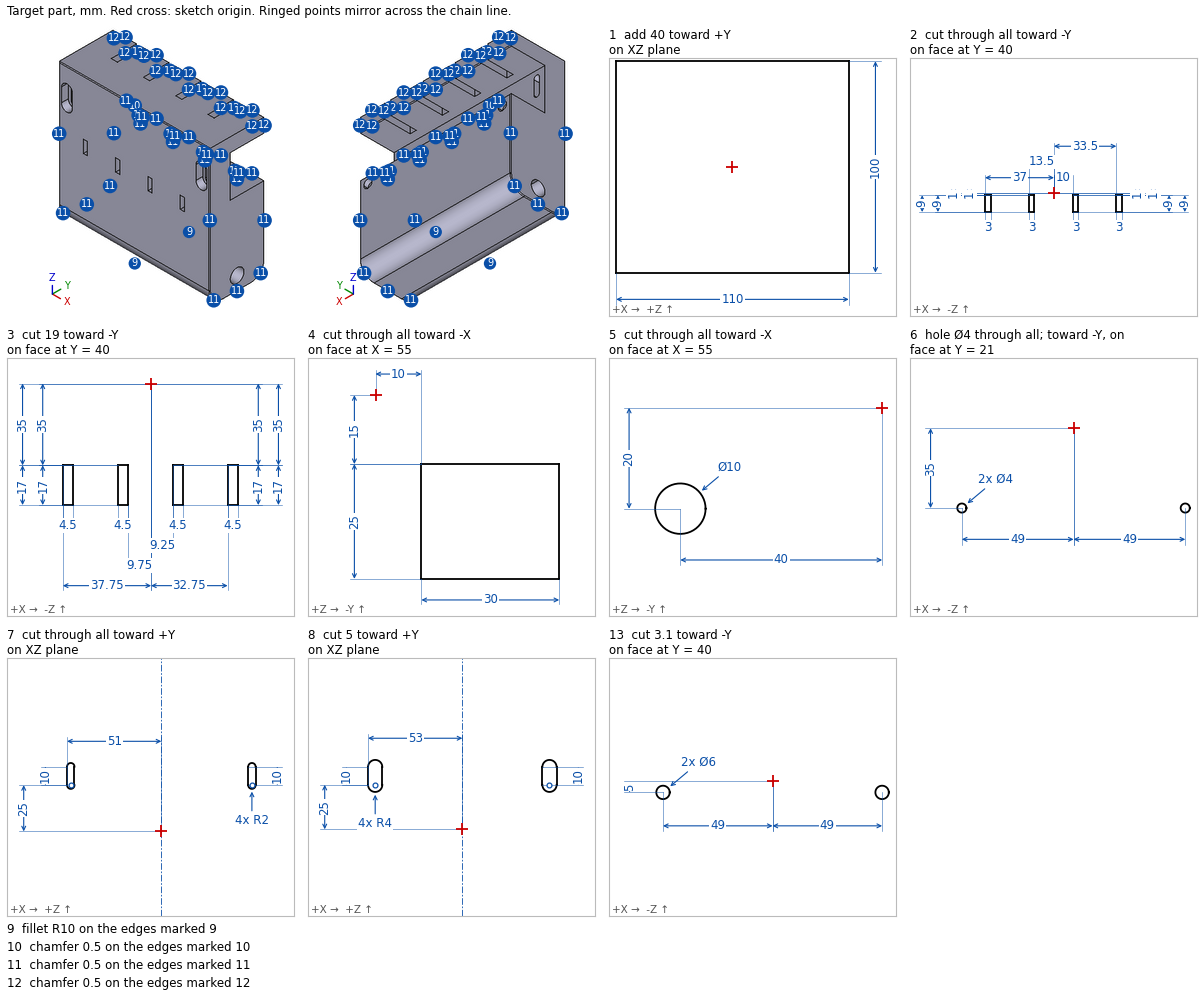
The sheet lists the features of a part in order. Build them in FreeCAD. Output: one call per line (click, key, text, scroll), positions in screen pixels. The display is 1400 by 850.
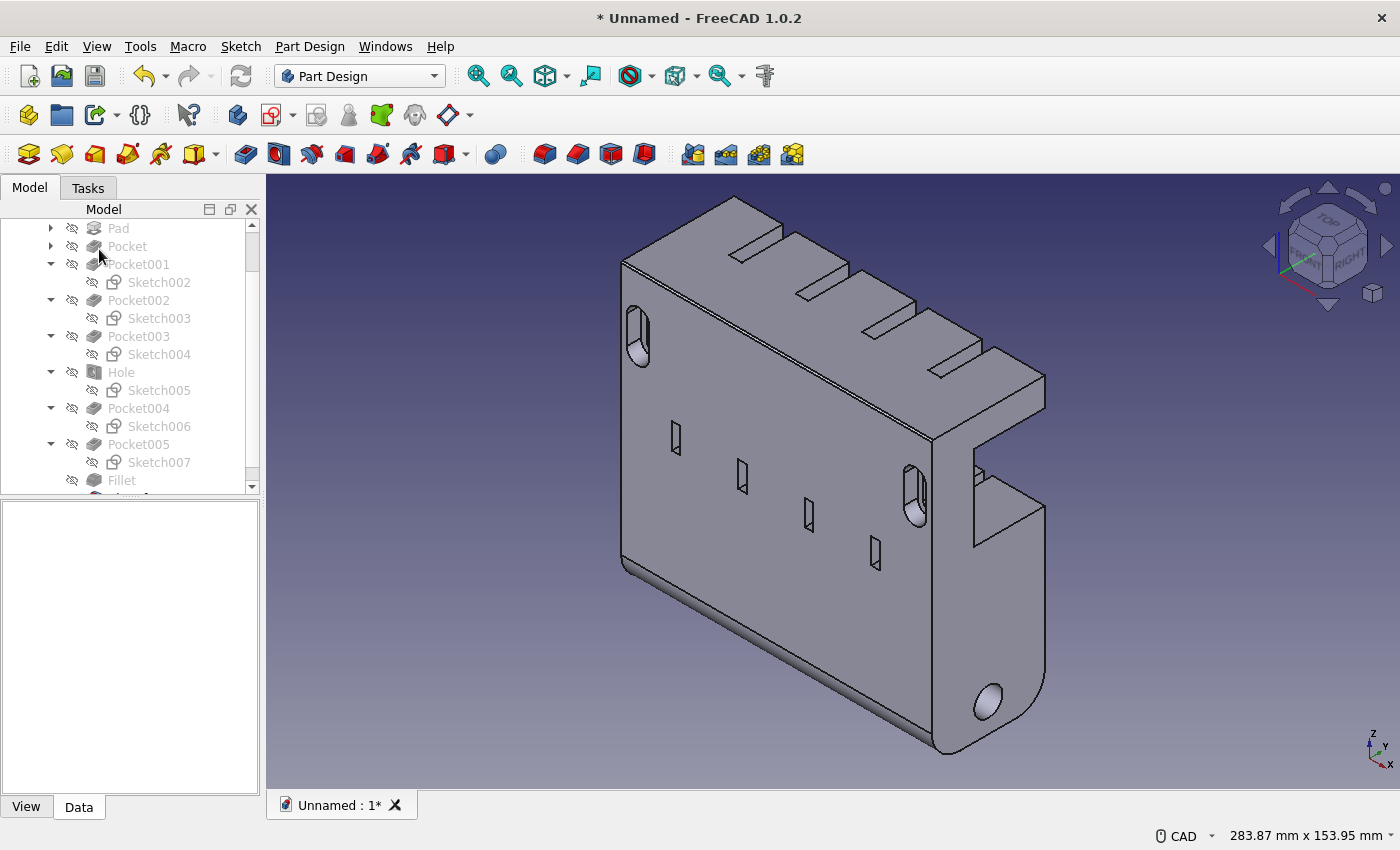
click(932, 587)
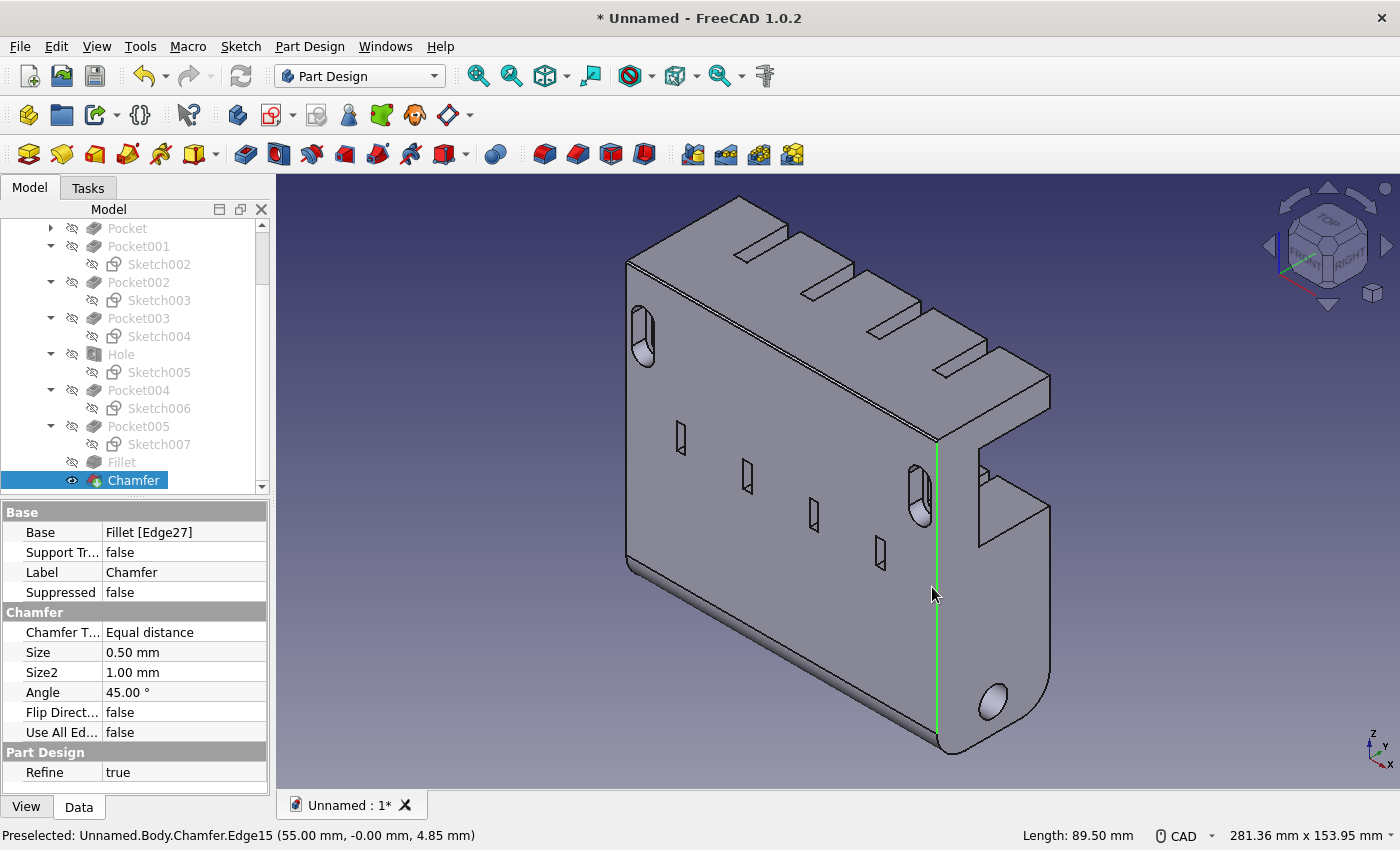
click(945, 752, ctrl)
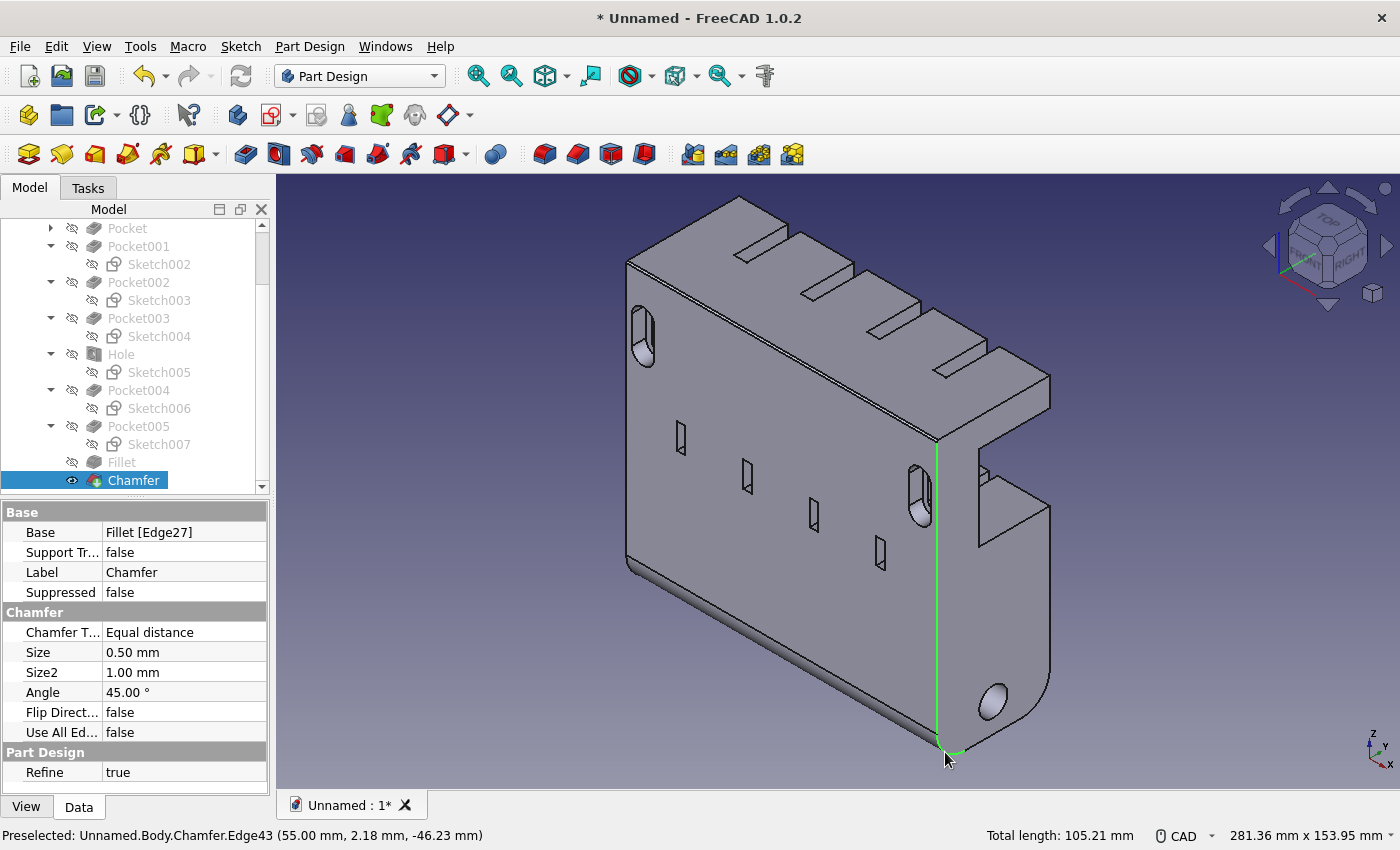
key(2)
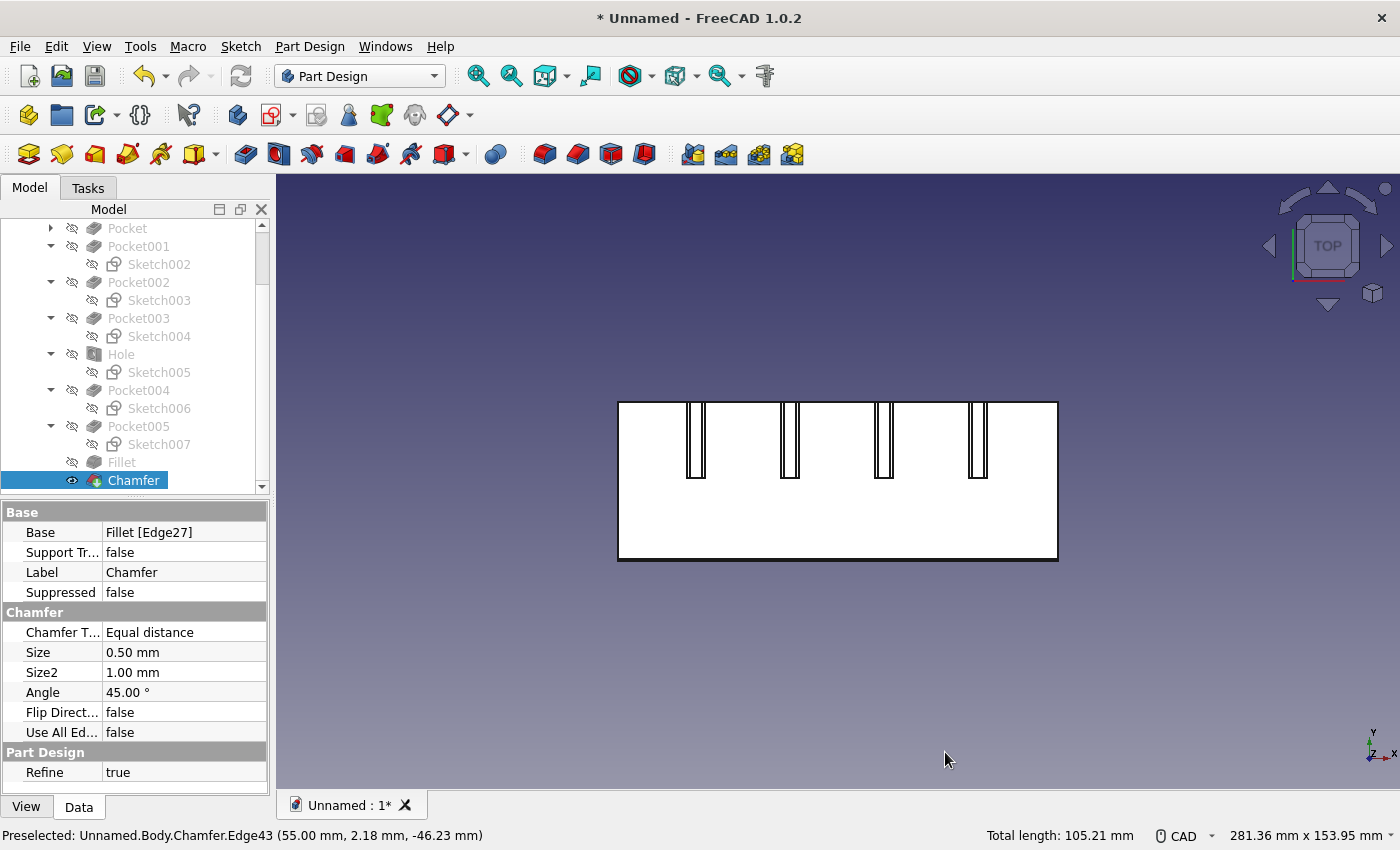
key(v)
key(f)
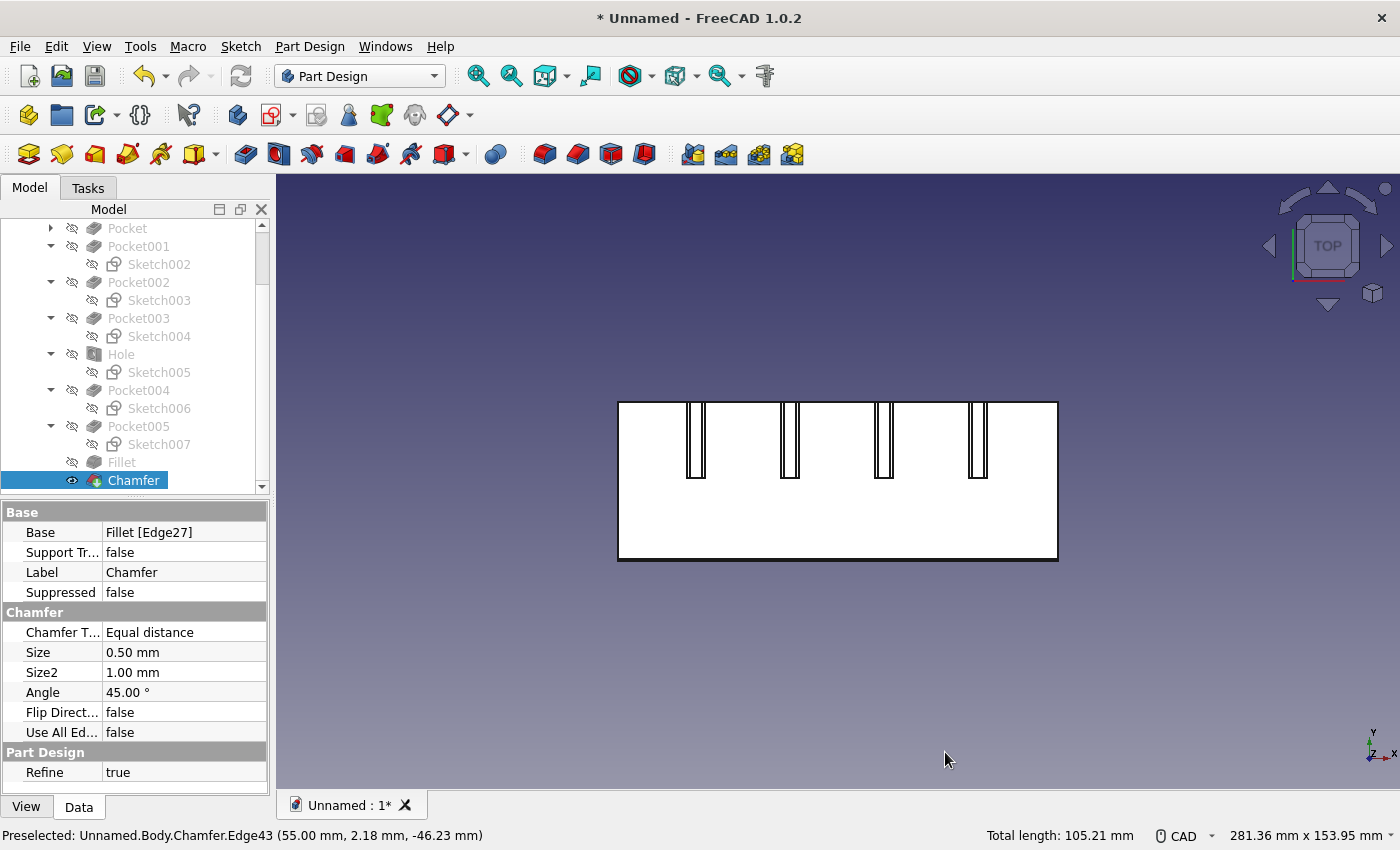
key(0)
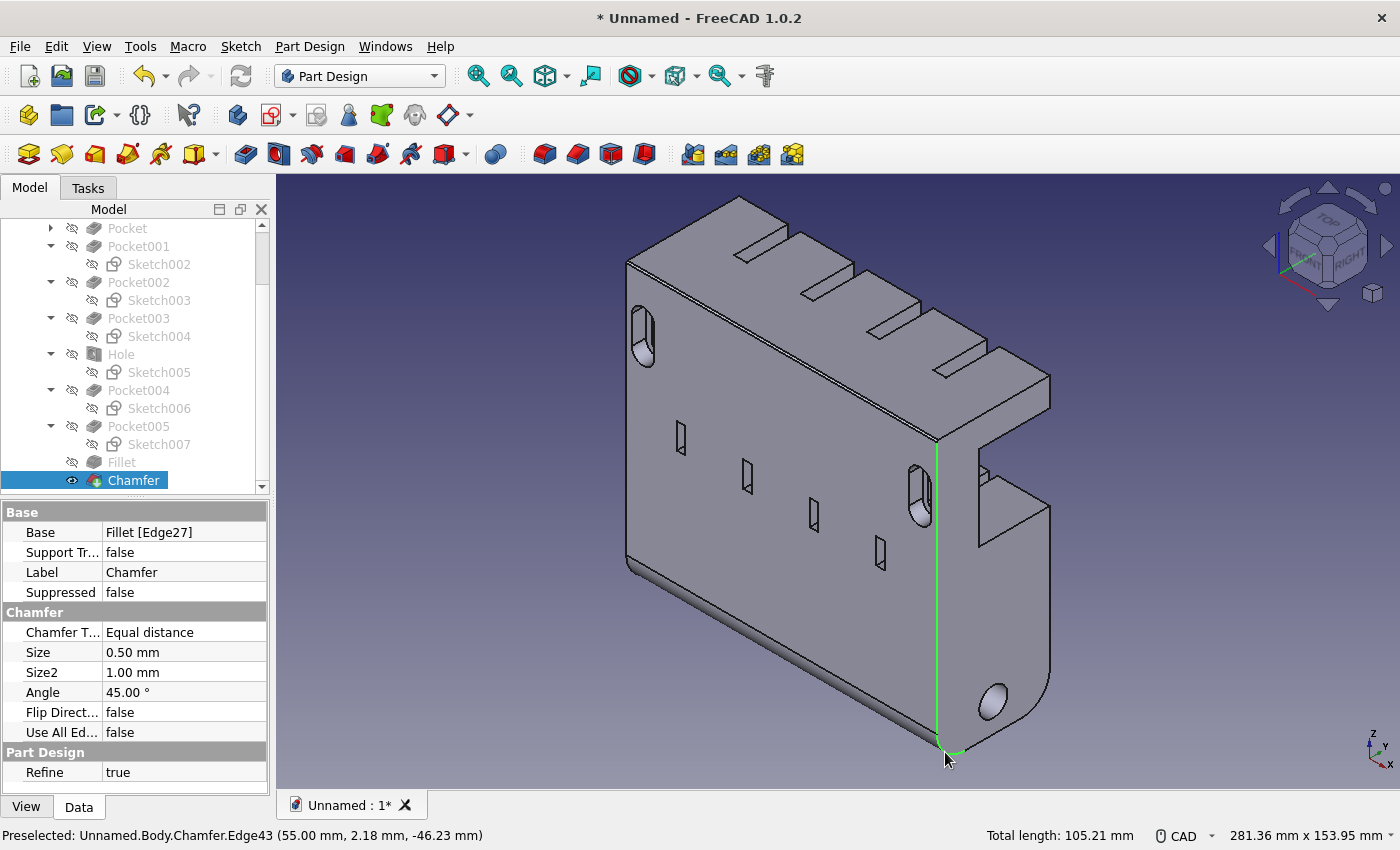
key(1)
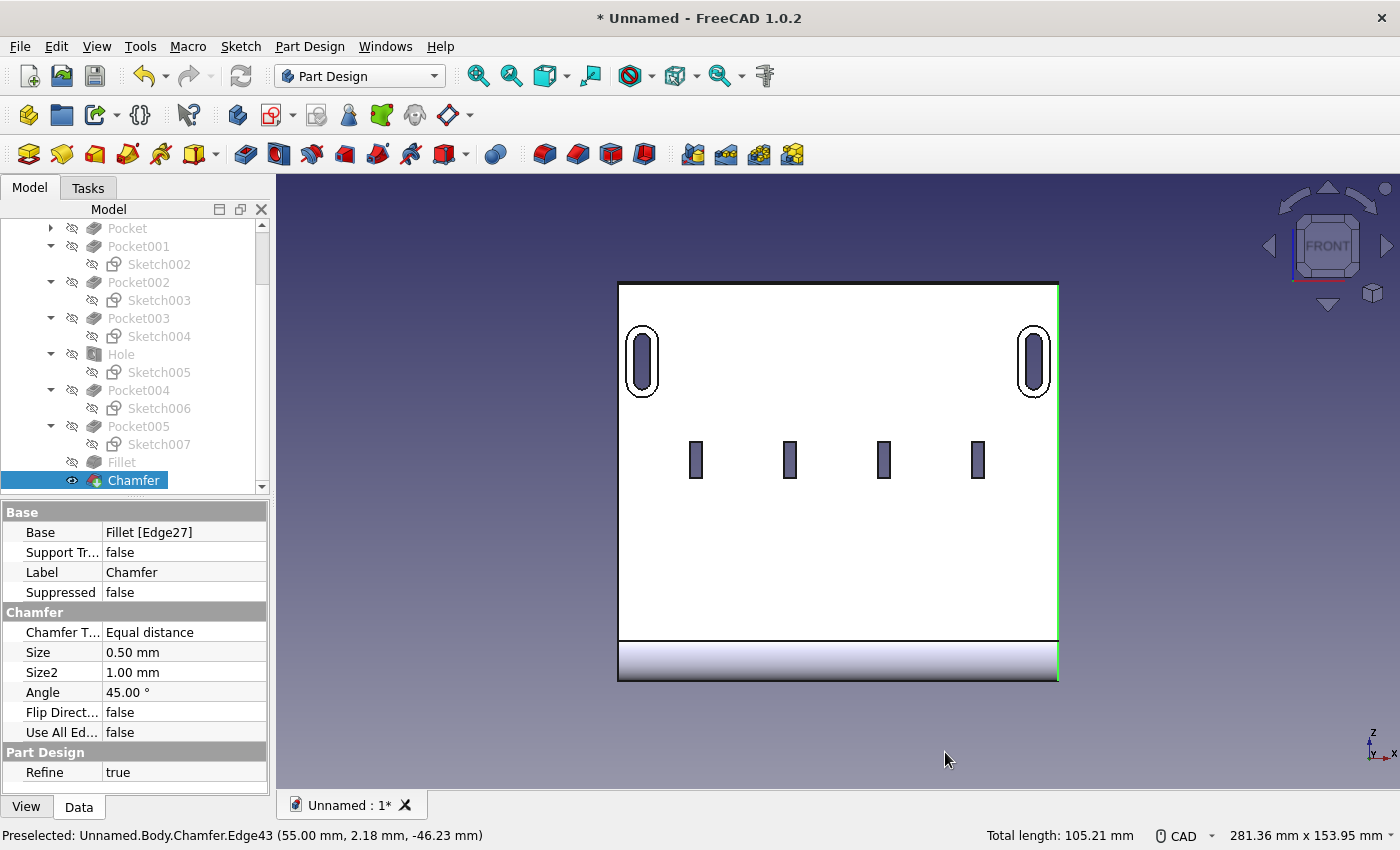
click(618, 462, ctrl)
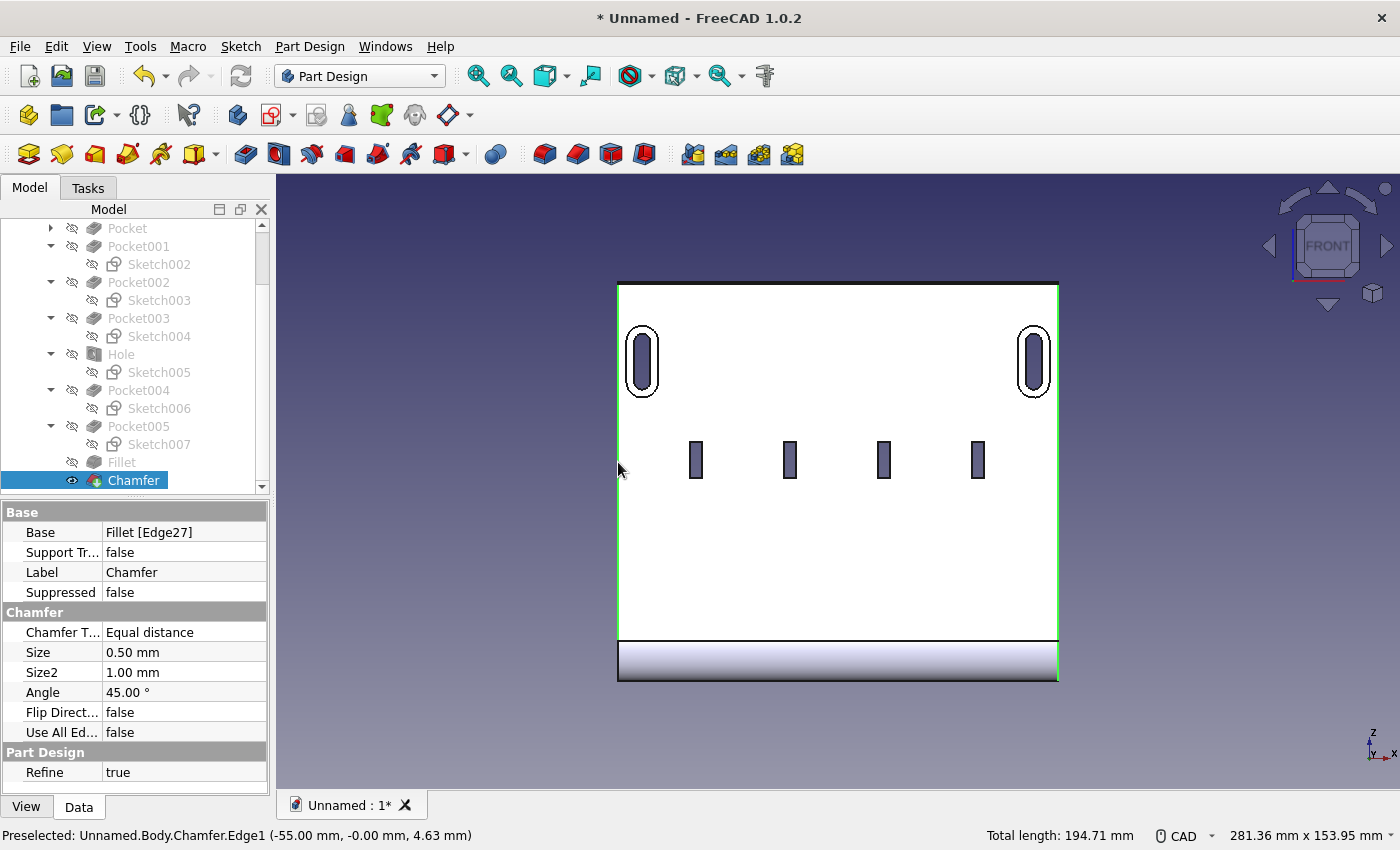
click(618, 669, ctrl)